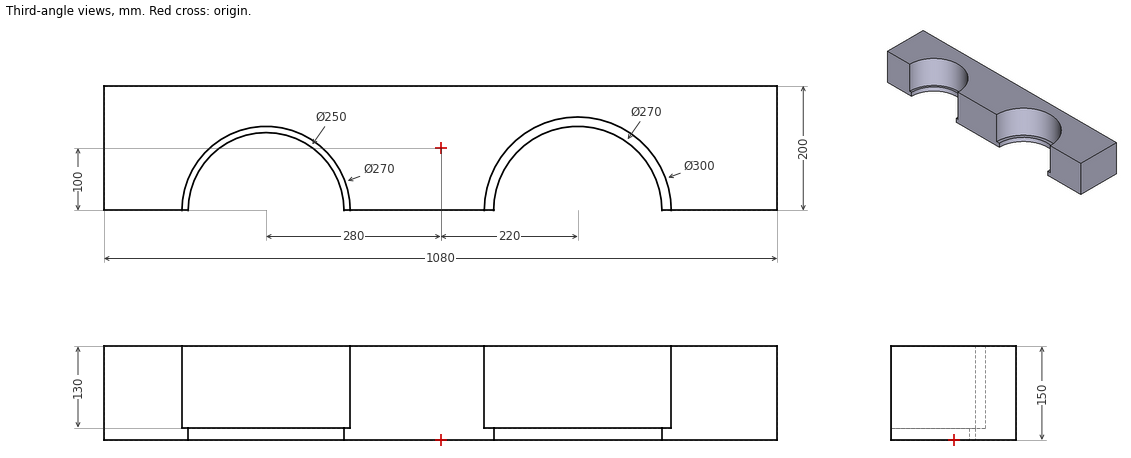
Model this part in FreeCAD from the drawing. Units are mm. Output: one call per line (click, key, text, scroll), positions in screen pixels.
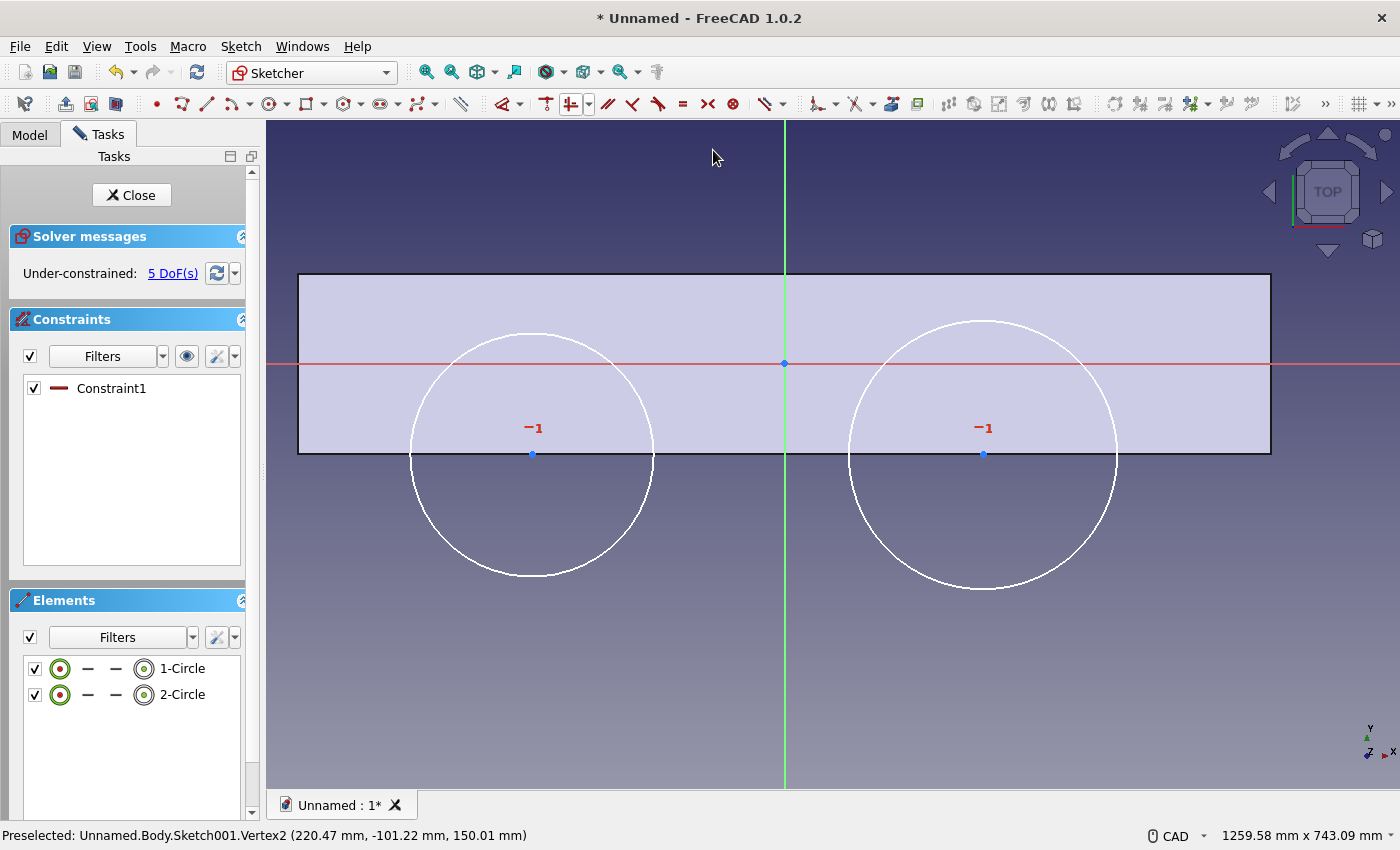
key(d)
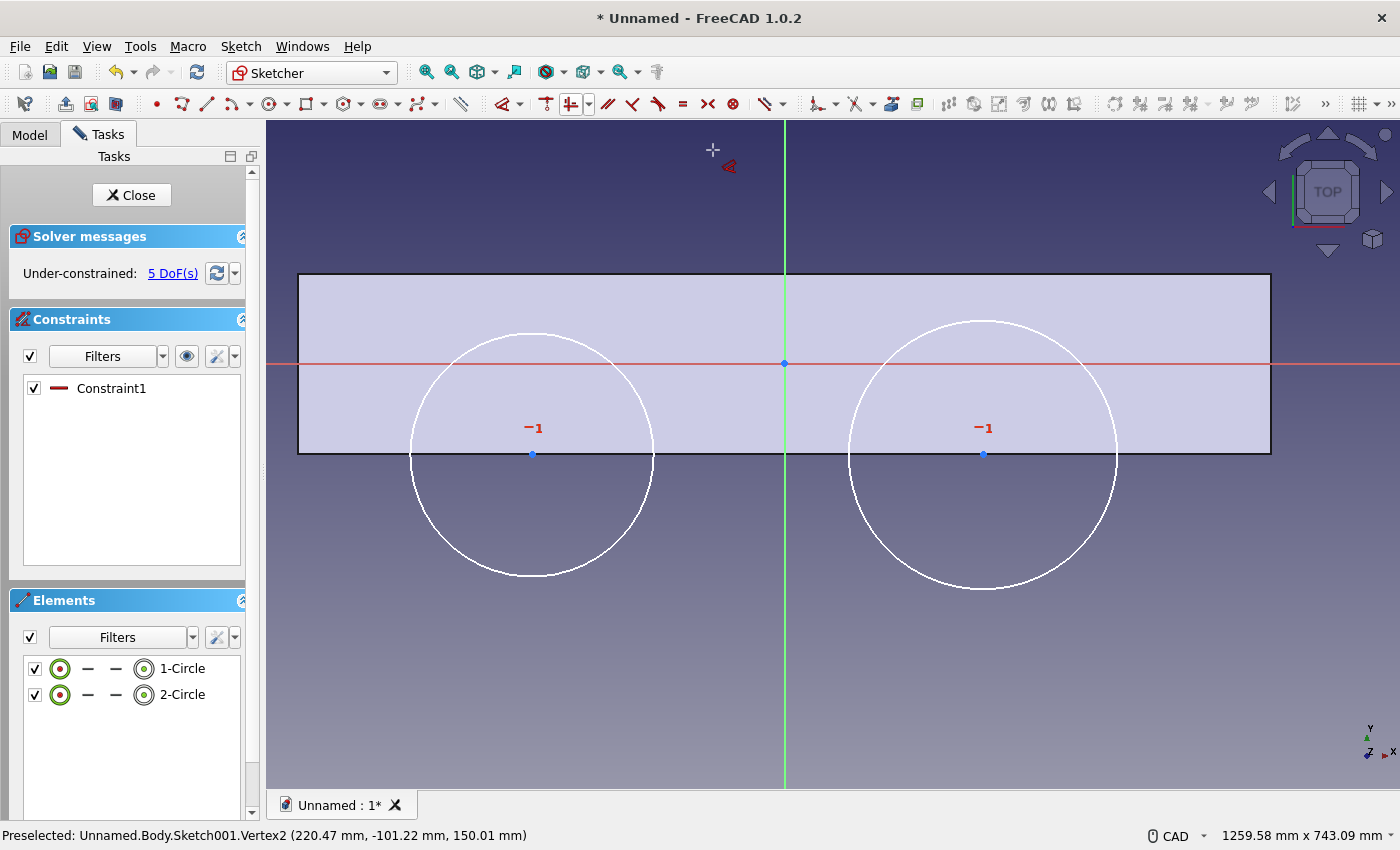
click(446, 541)
click(423, 564)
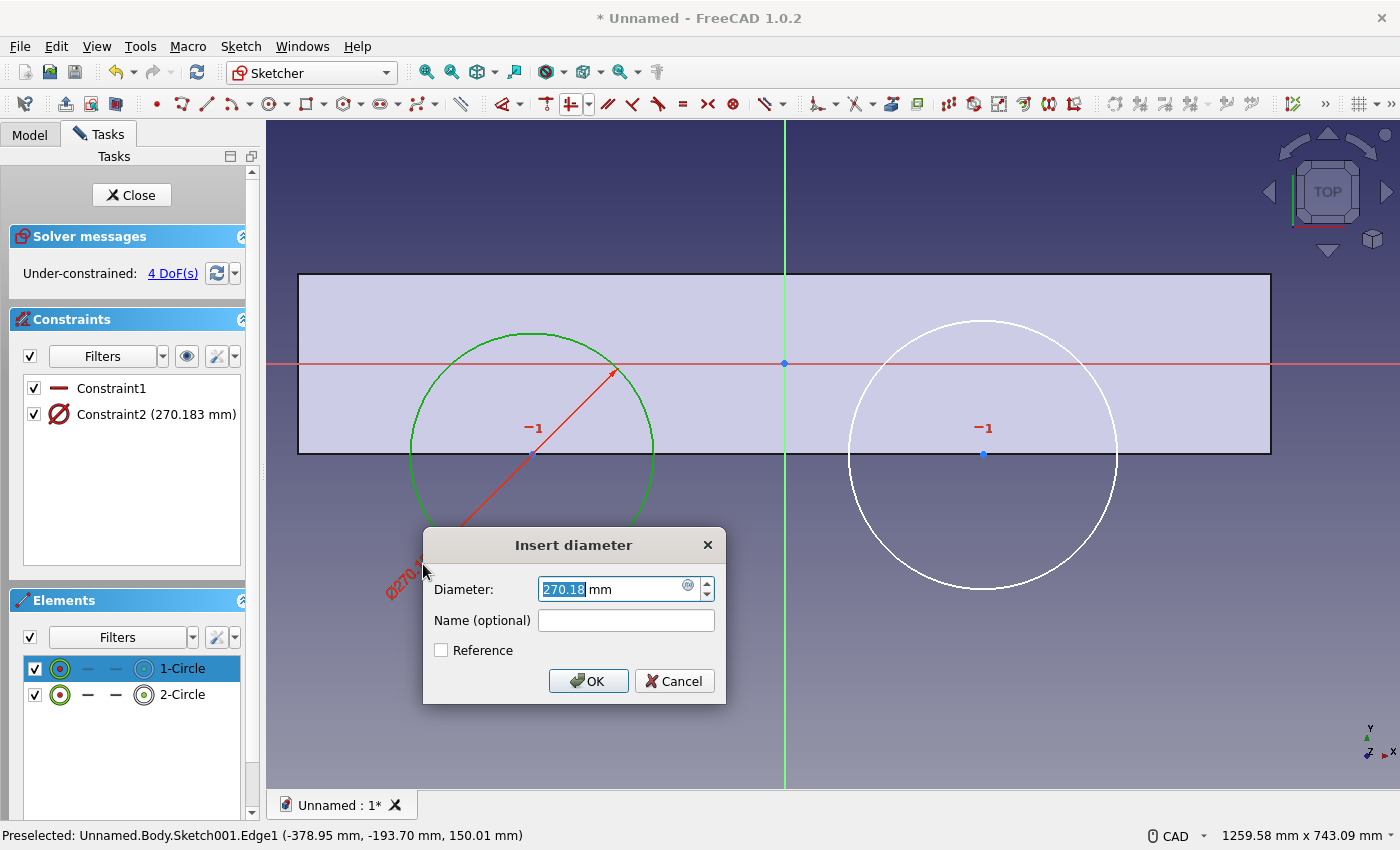
text(270)
key(Return)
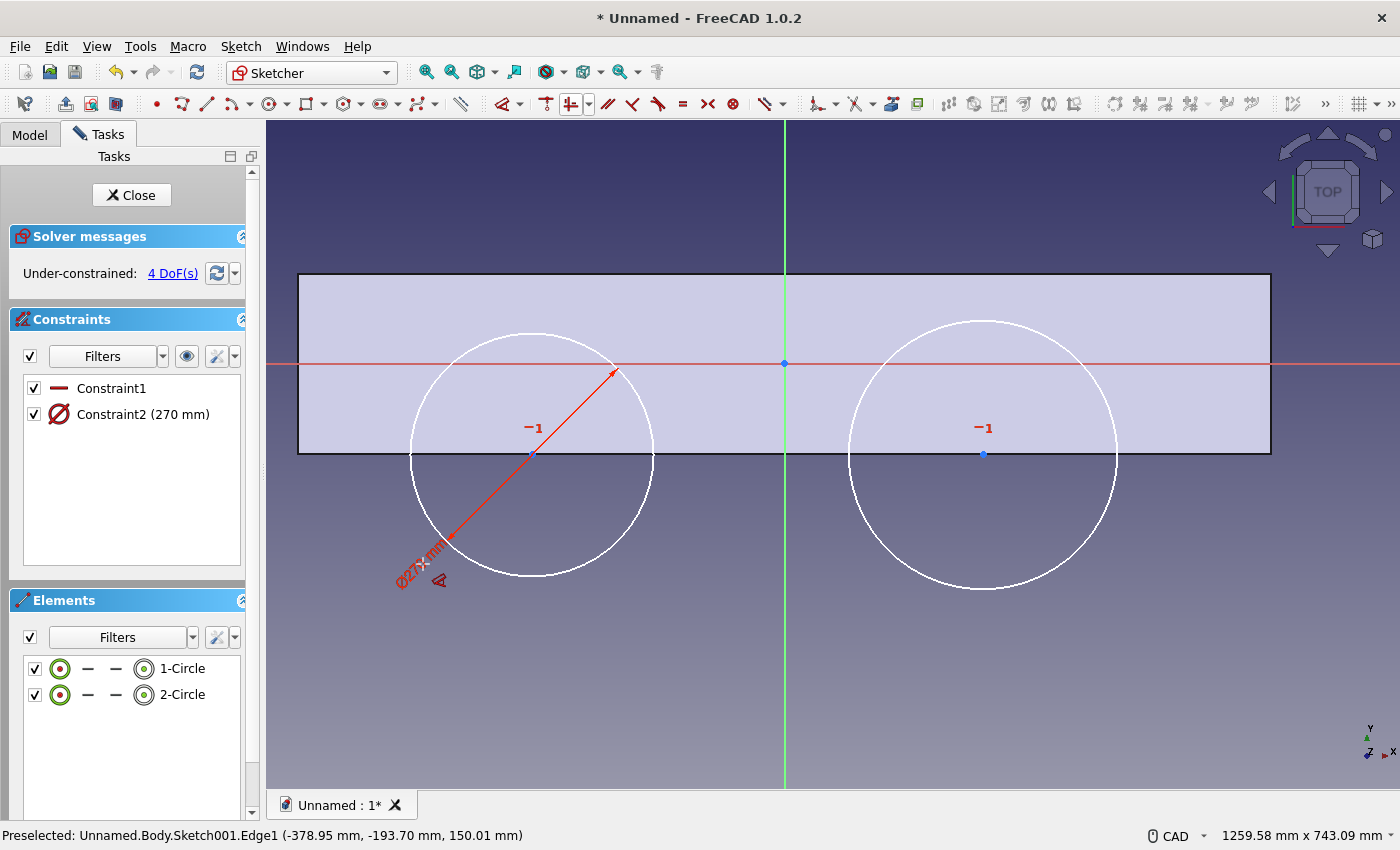
click(888, 360)
click(865, 337)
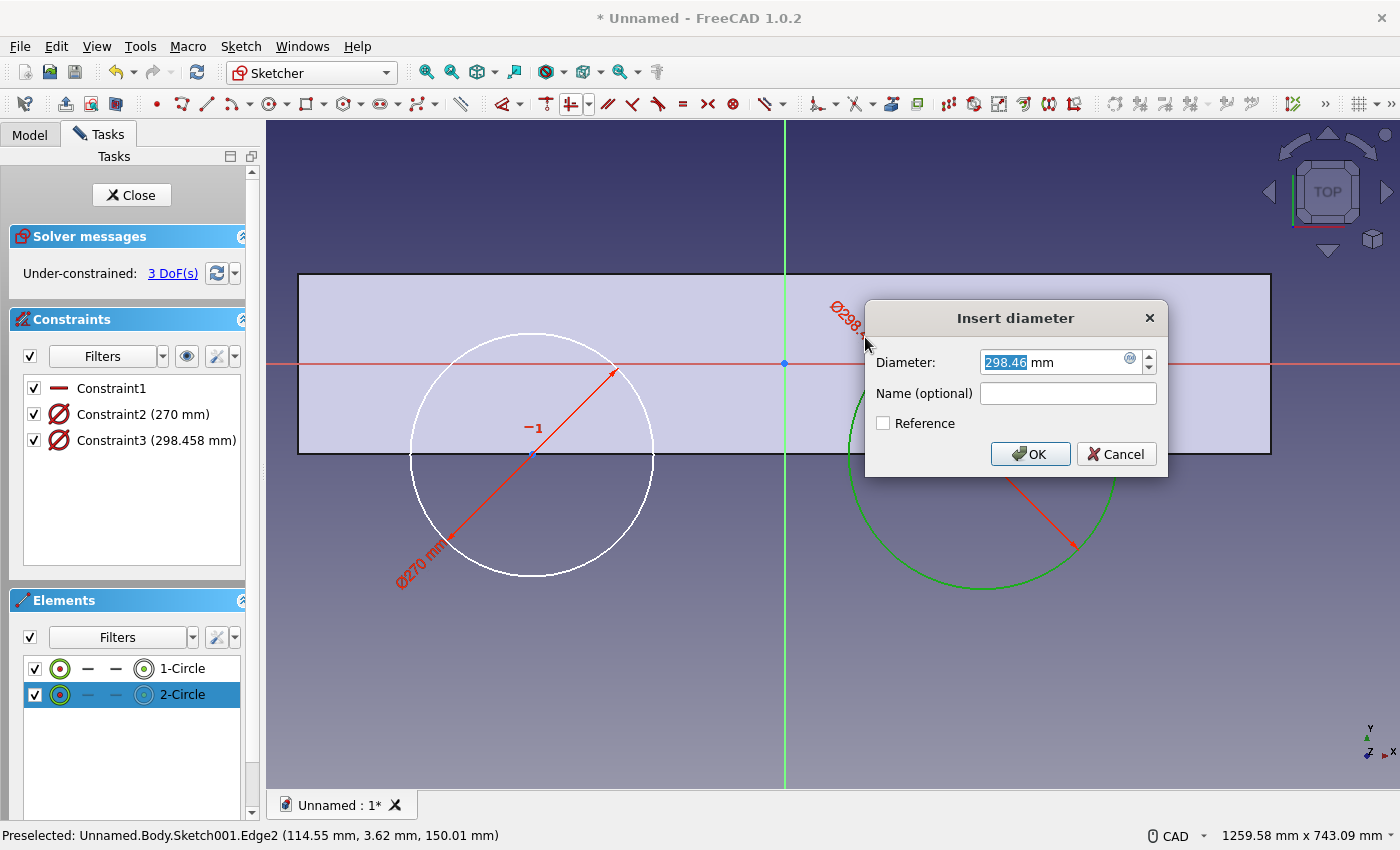
text(300)
key(Return)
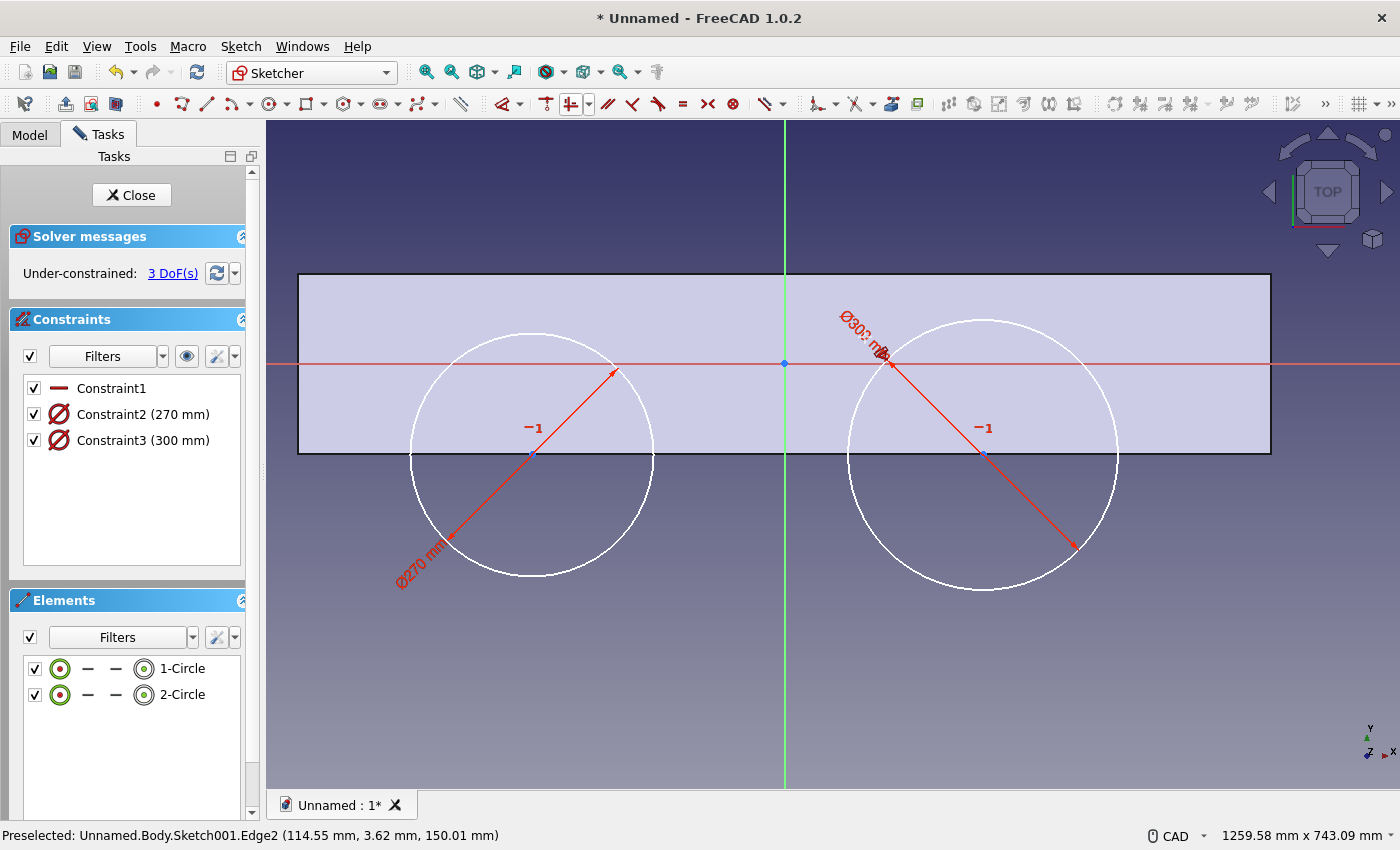
click(532, 455)
click(658, 330)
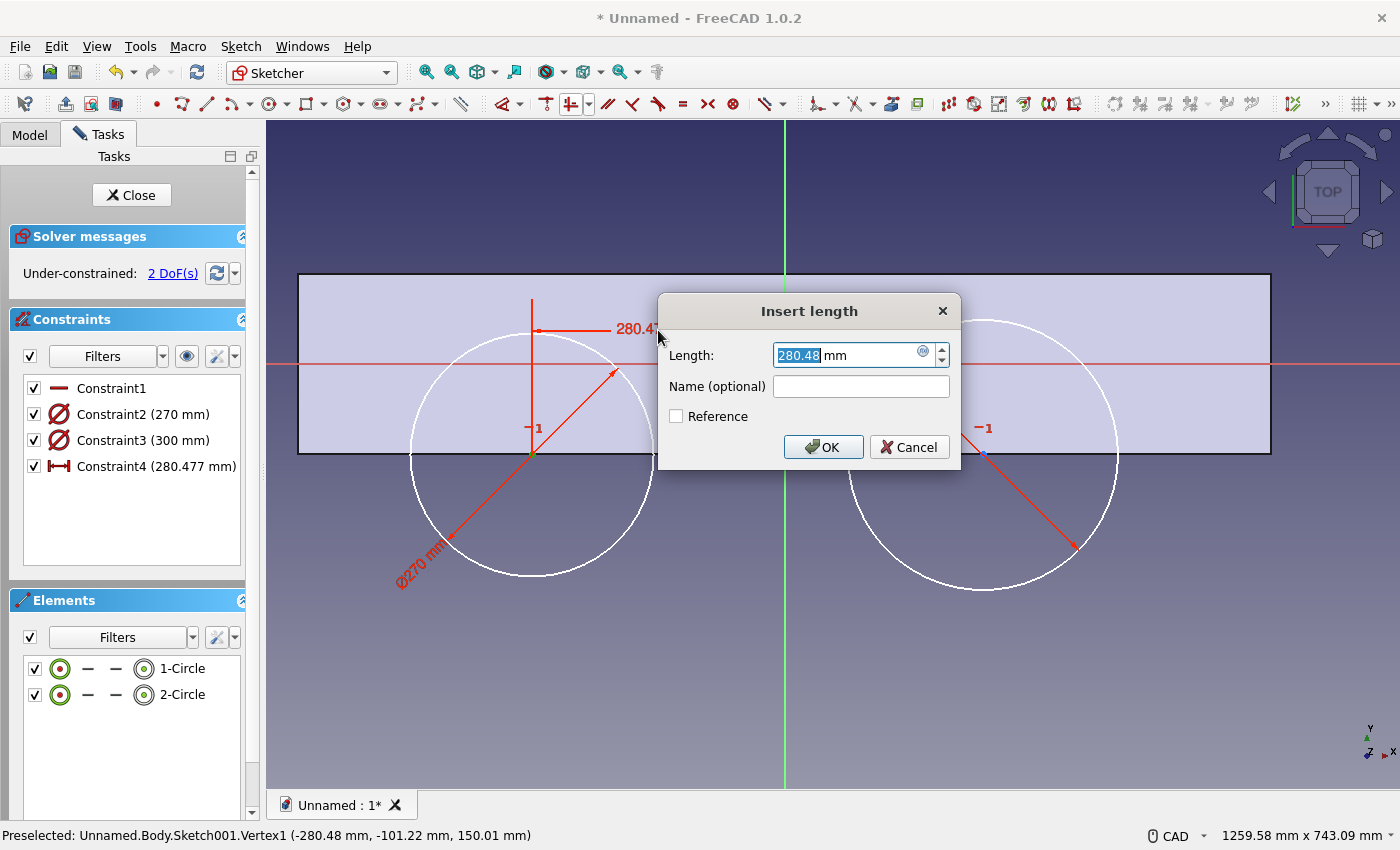
text(280)
key(Return)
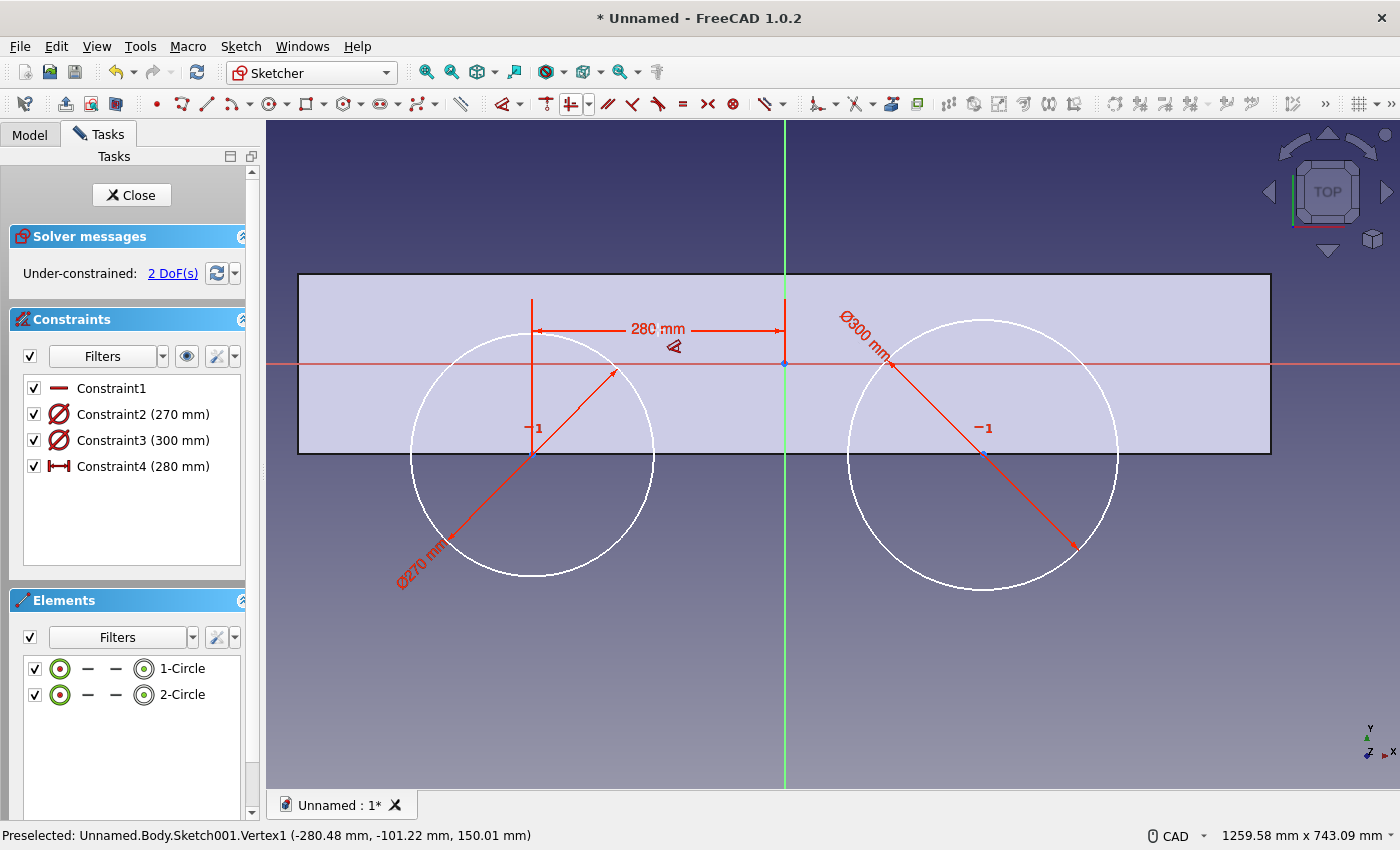
click(532, 455)
click(498, 409)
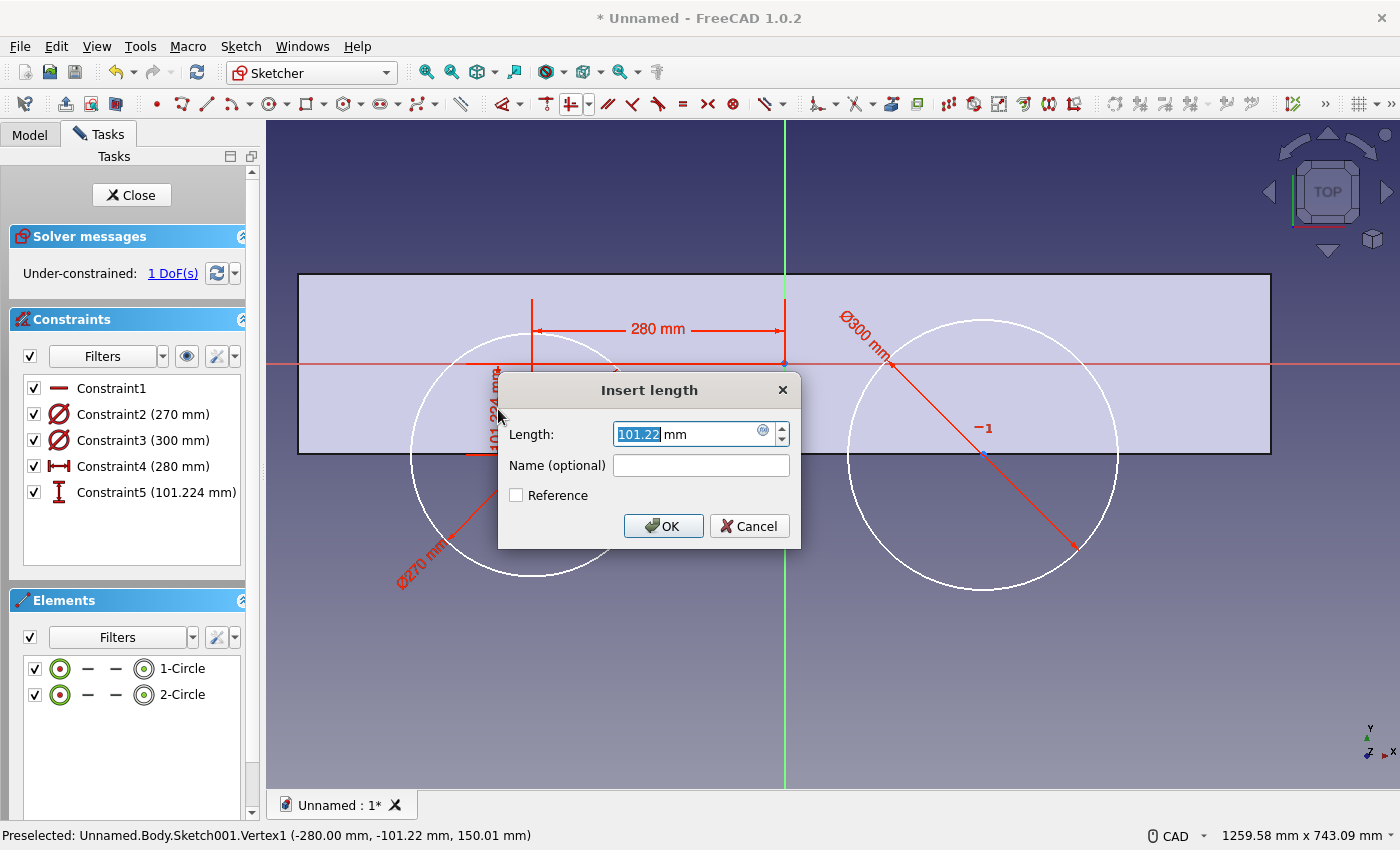
text(100)
key(Return)